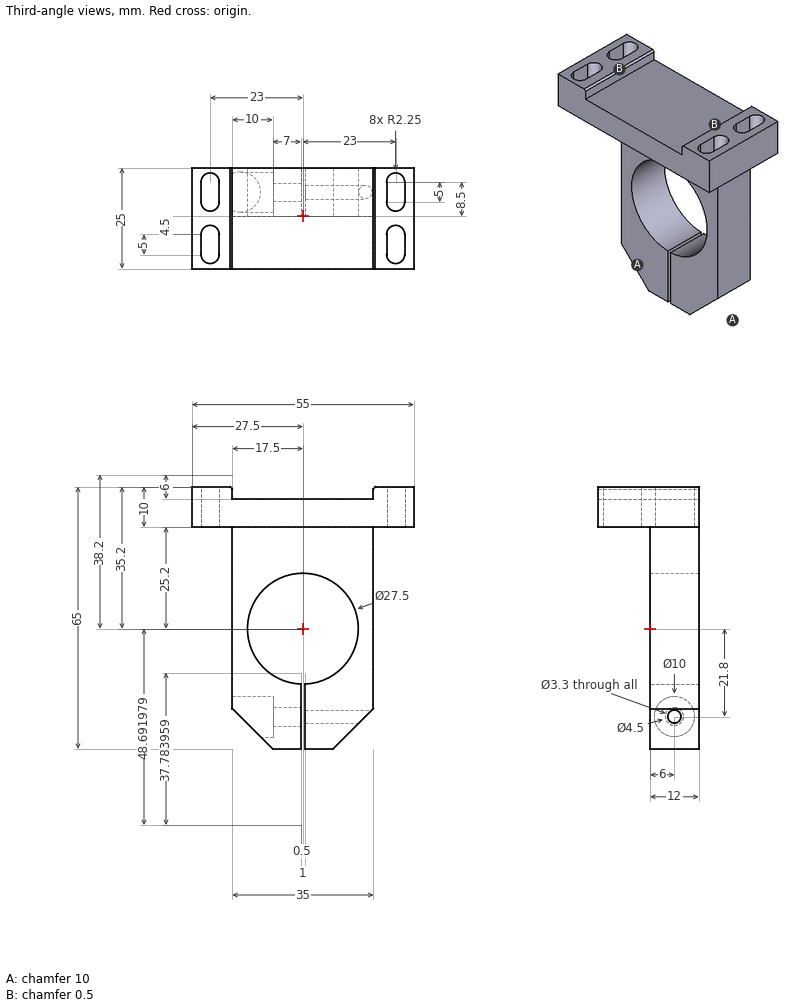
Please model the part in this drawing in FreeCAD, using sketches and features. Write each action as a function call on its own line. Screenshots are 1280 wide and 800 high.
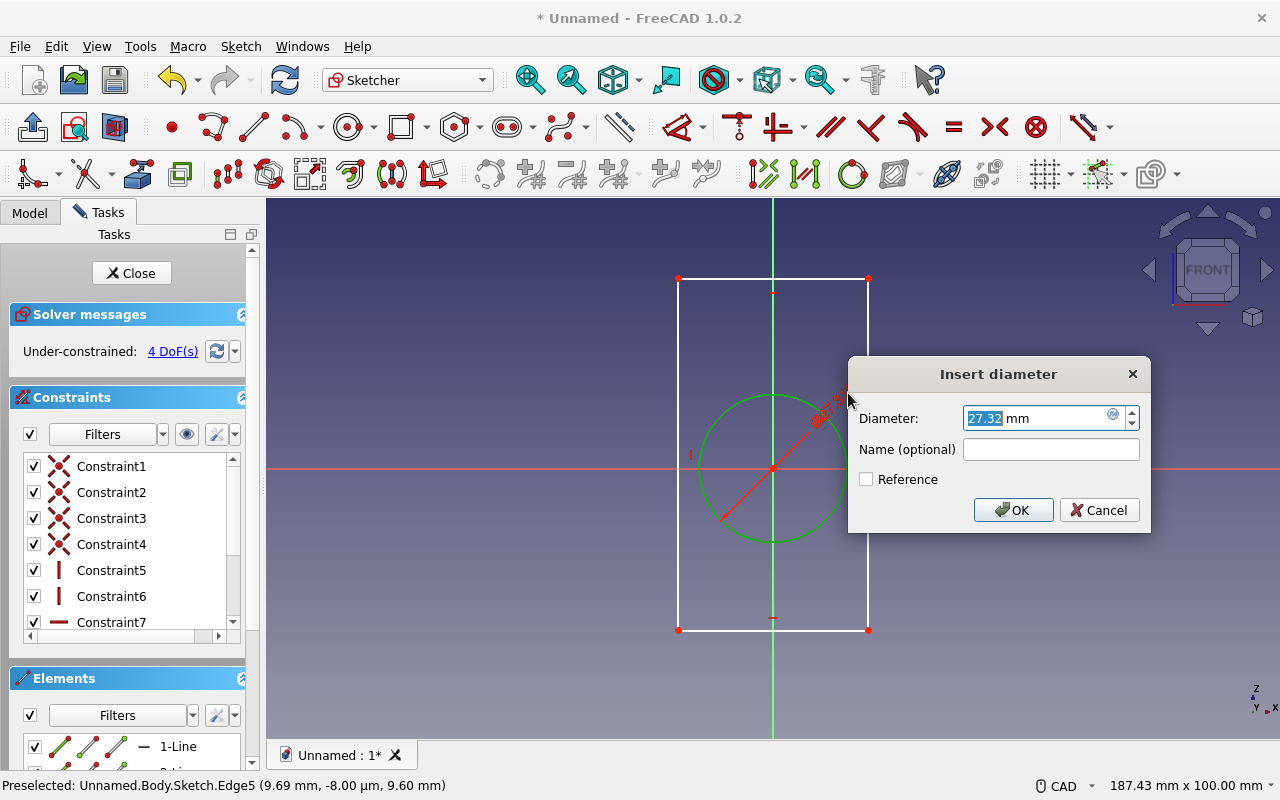
text(27.5)
key(Return)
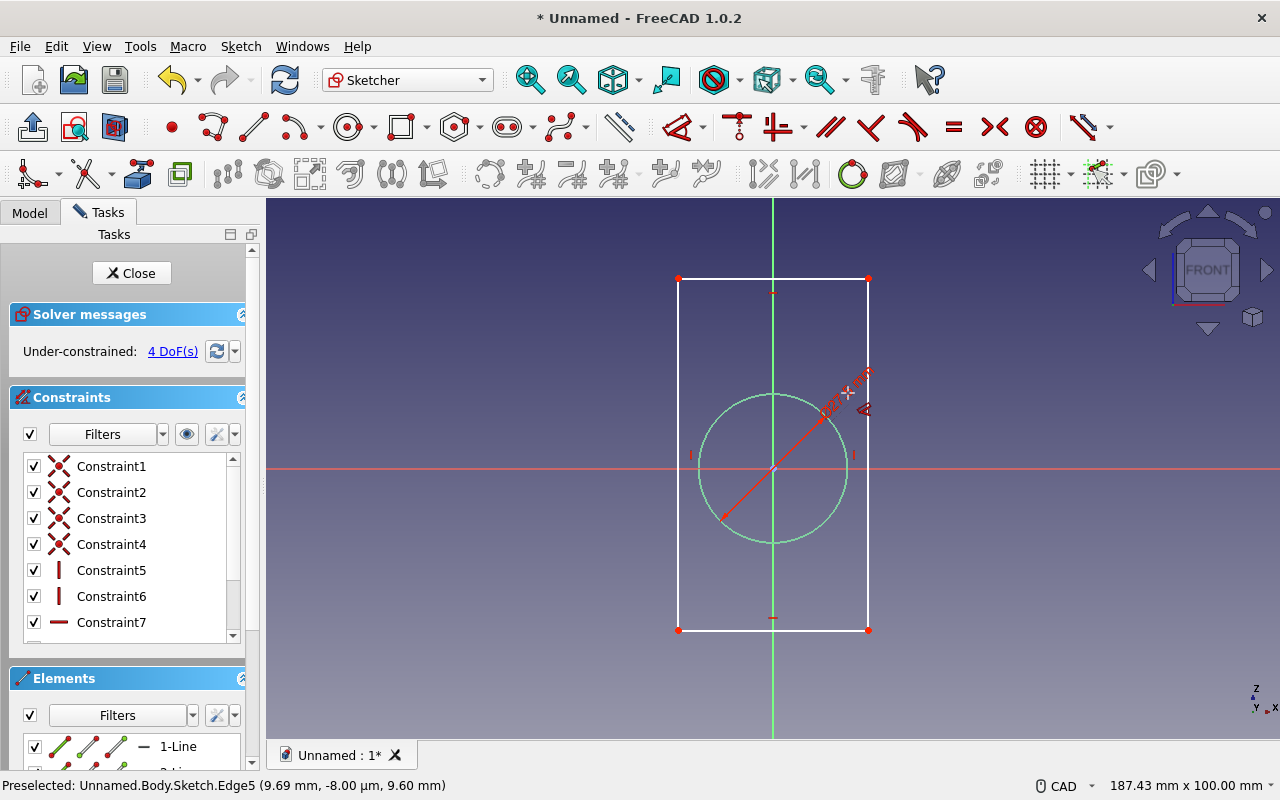
click(678, 385)
click(644, 455)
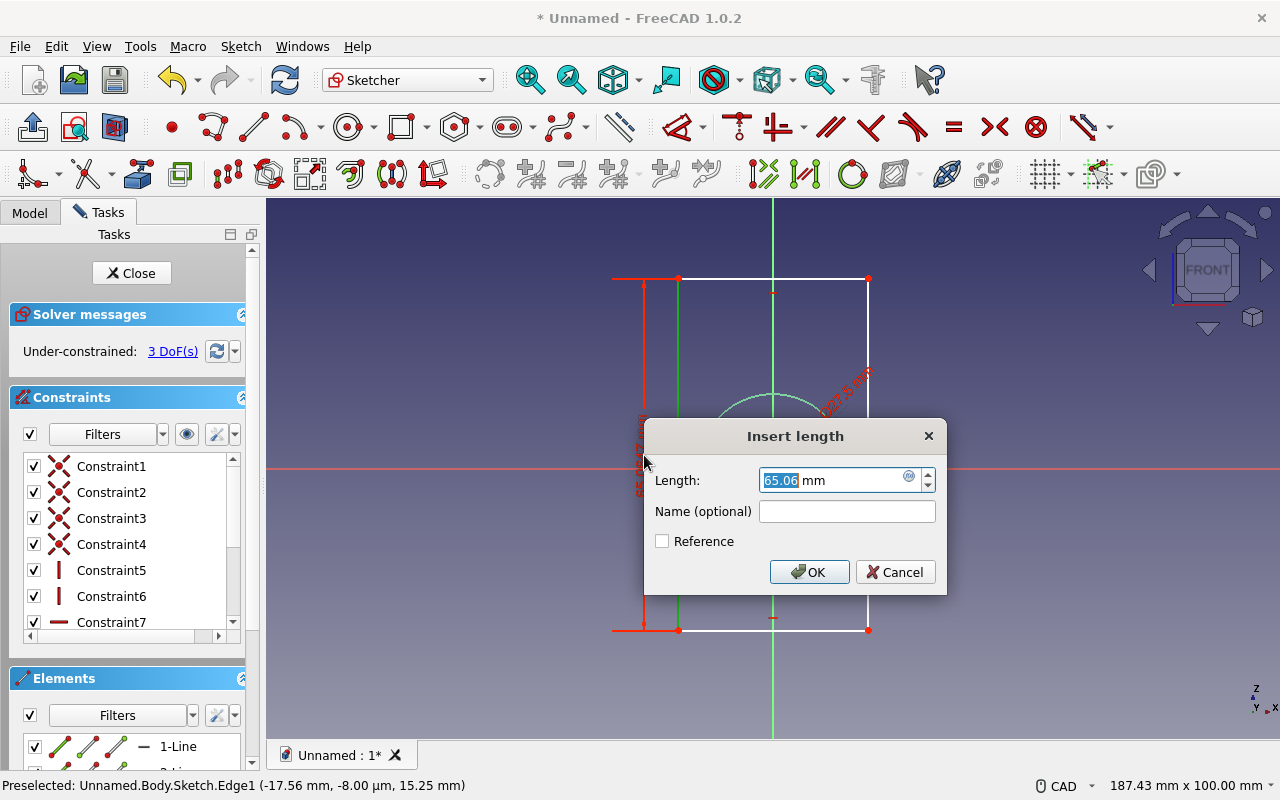
text(65)
key(Return)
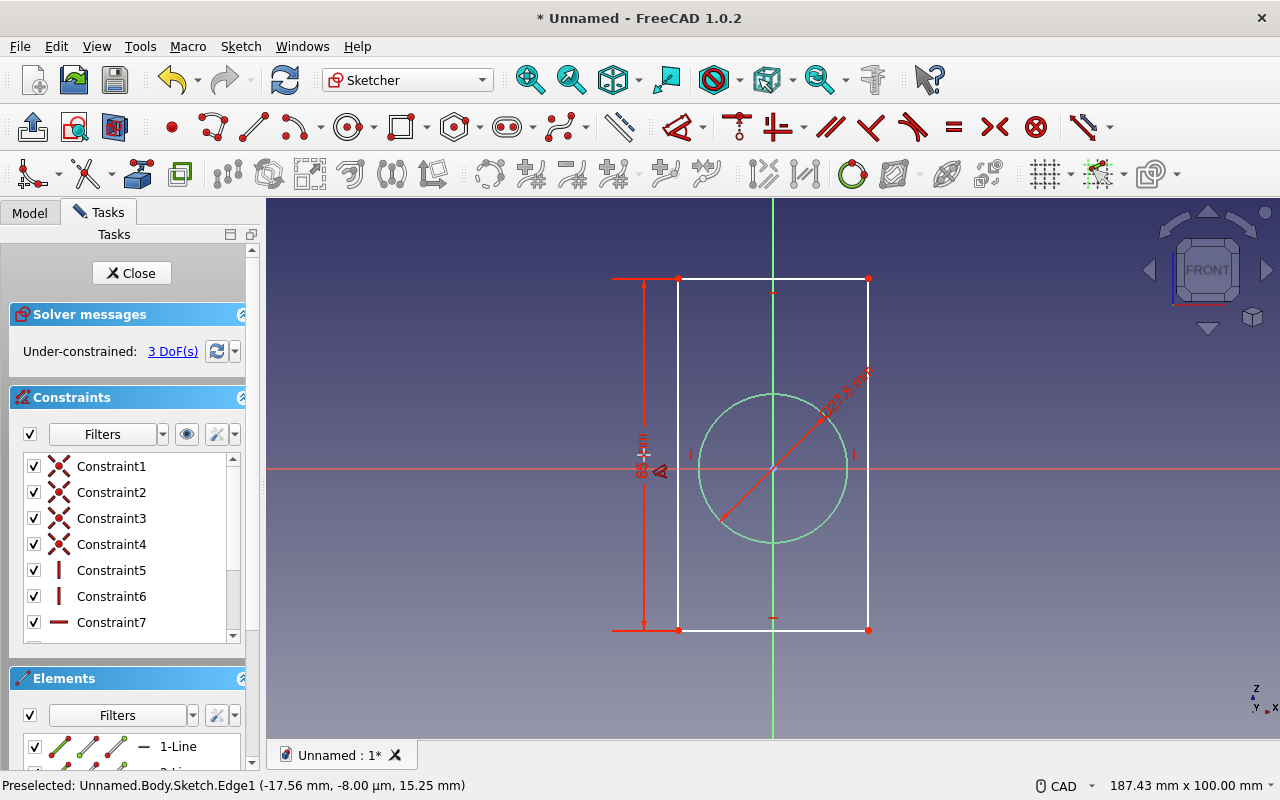
click(735, 631)
click(729, 665)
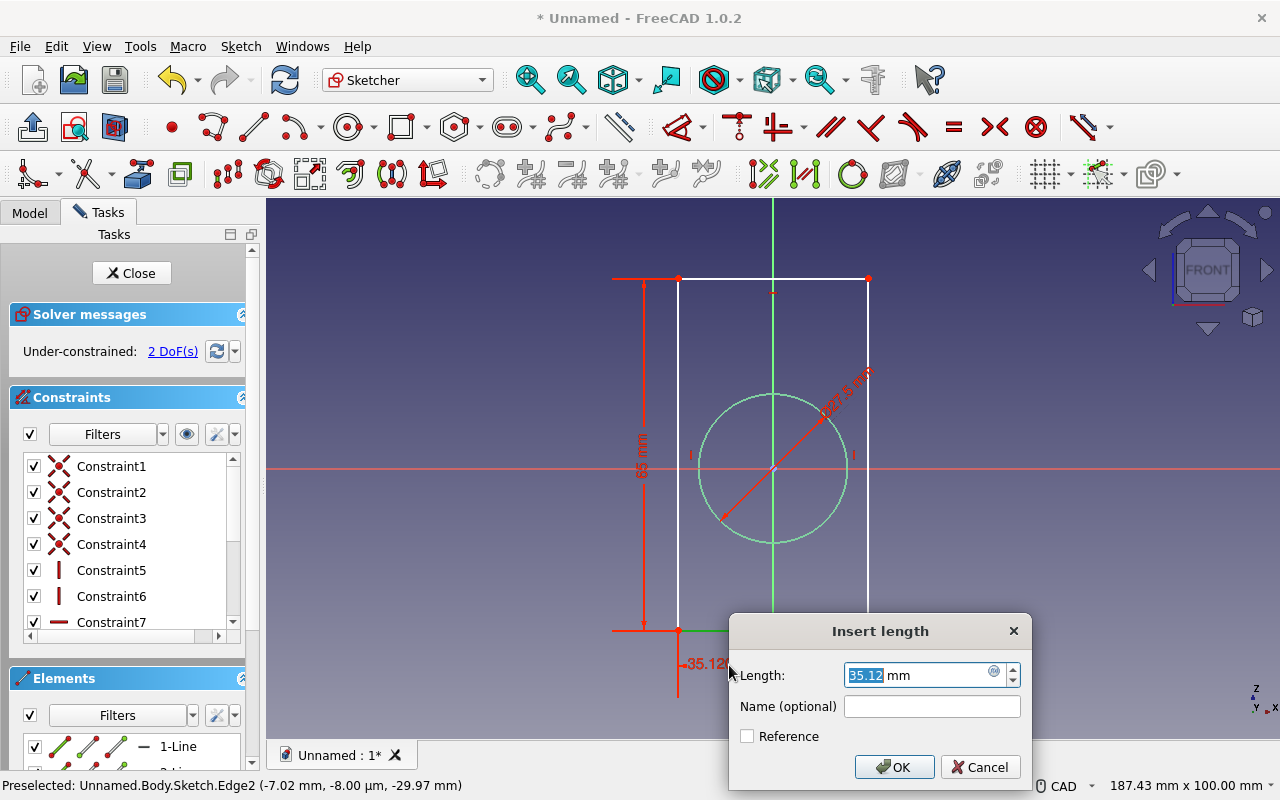
text(35)
key(Return)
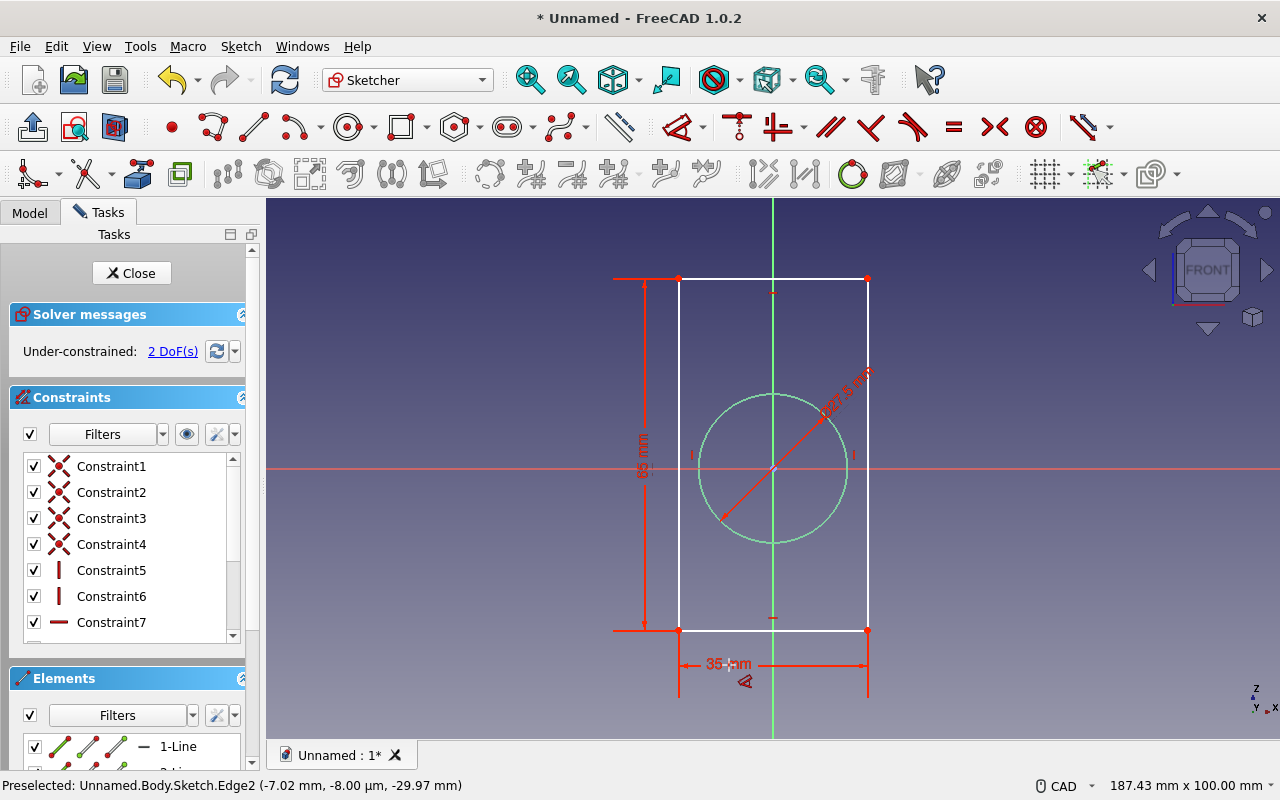
click(679, 279)
click(726, 245)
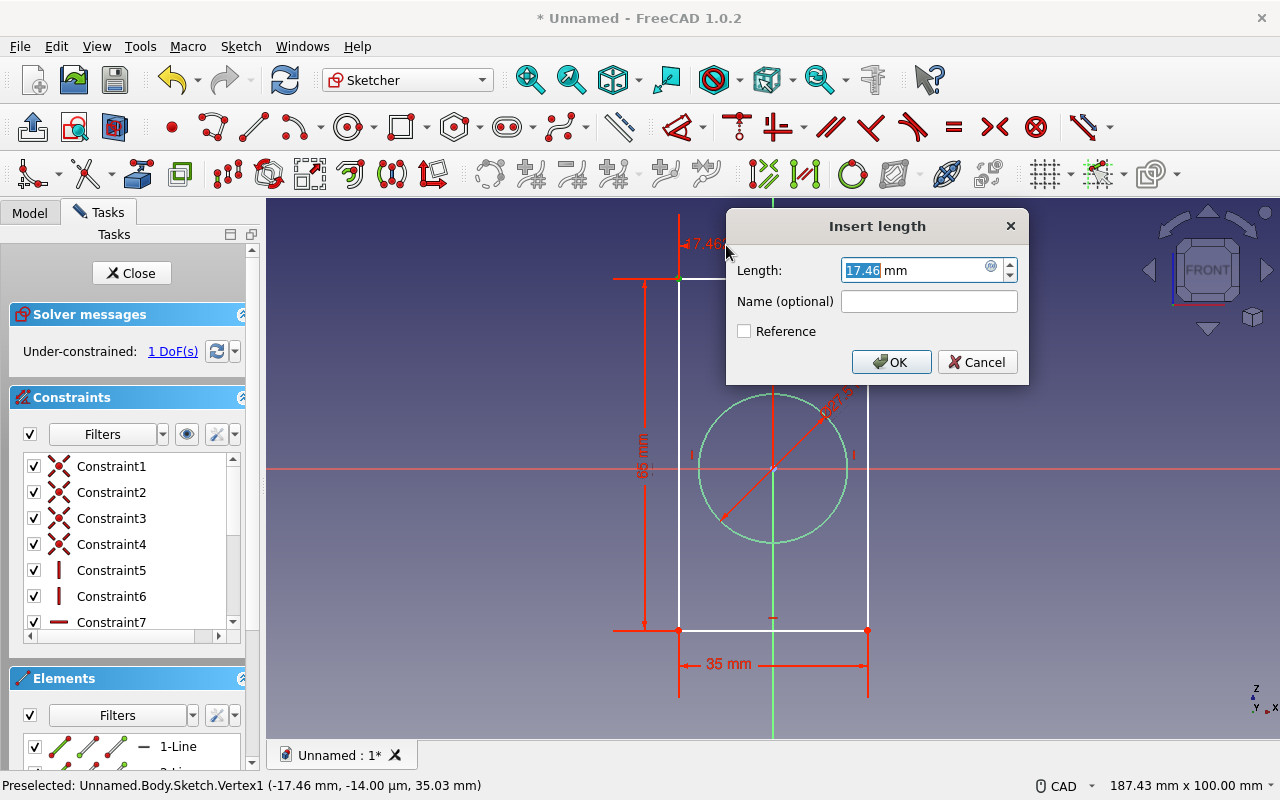
text(17.5)
key(Return)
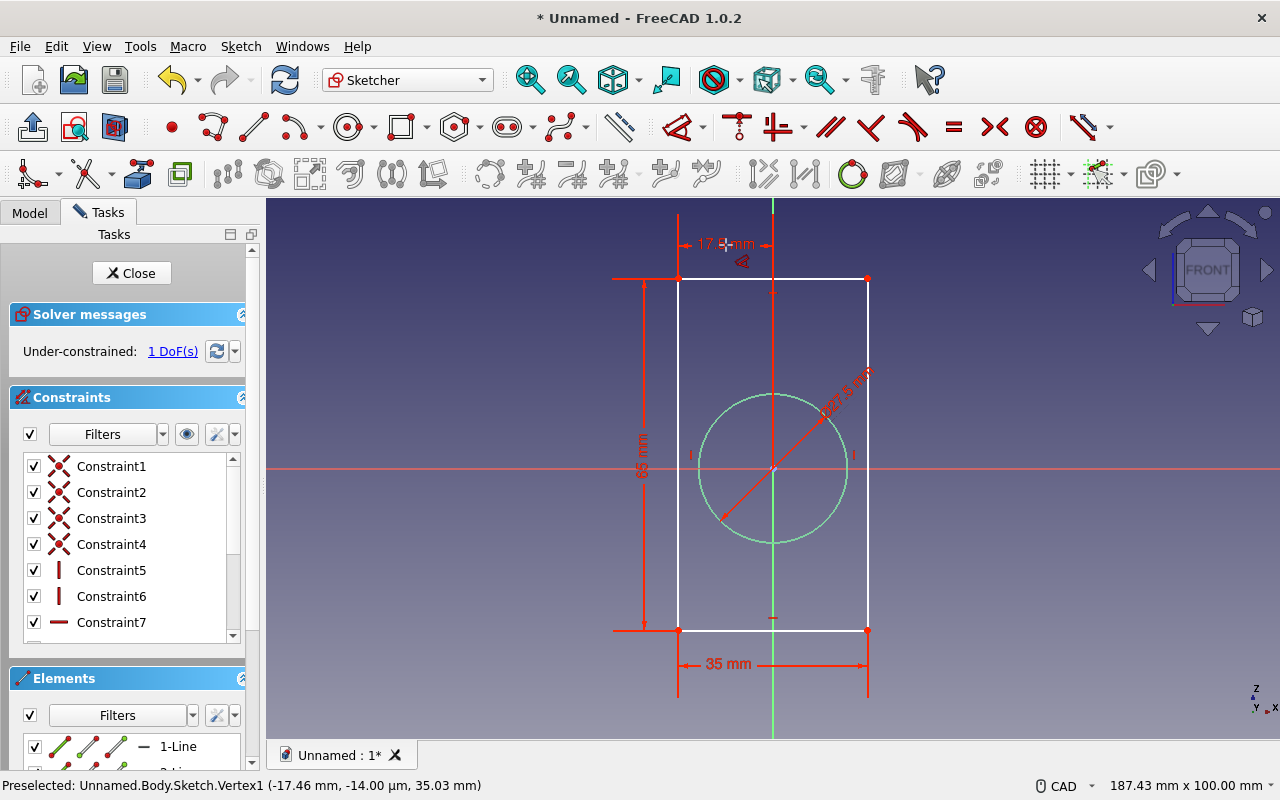
click(678, 279)
click(644, 374)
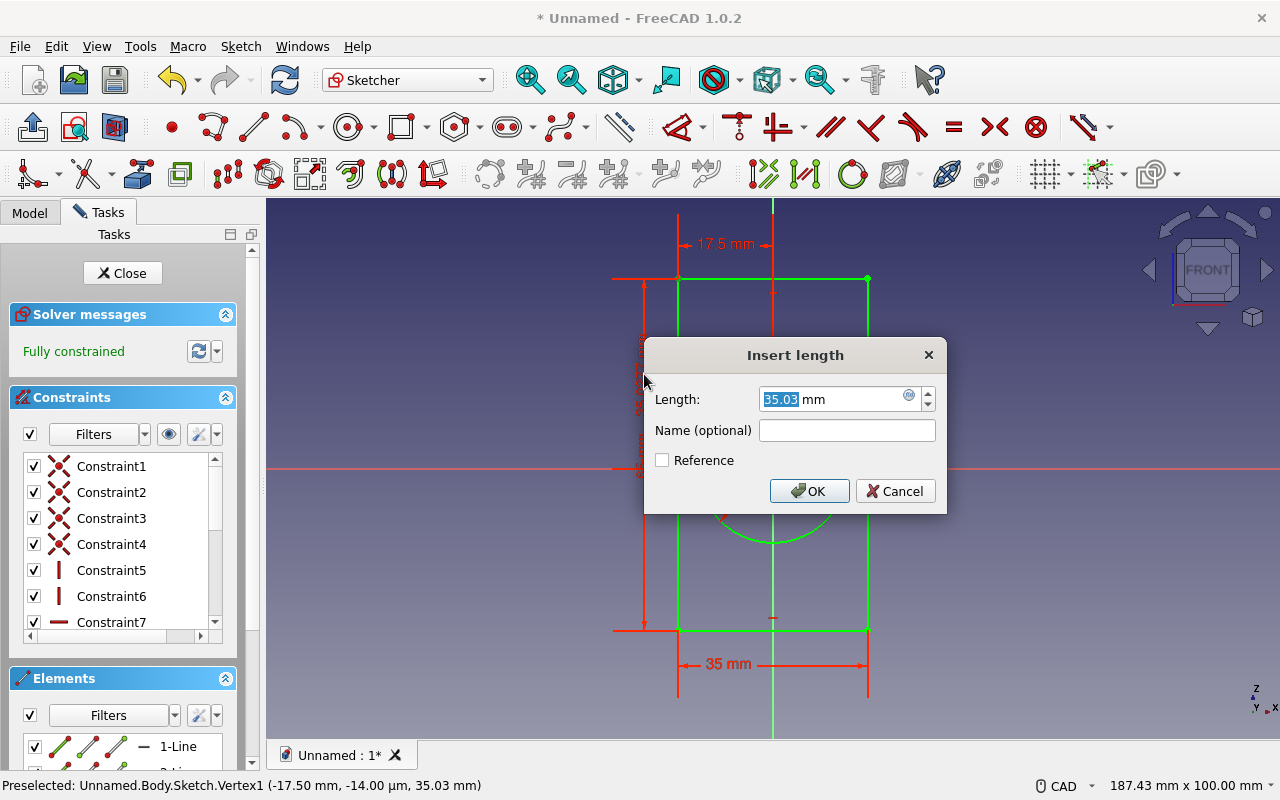
text(35.2)
key(Return)
key(Escape)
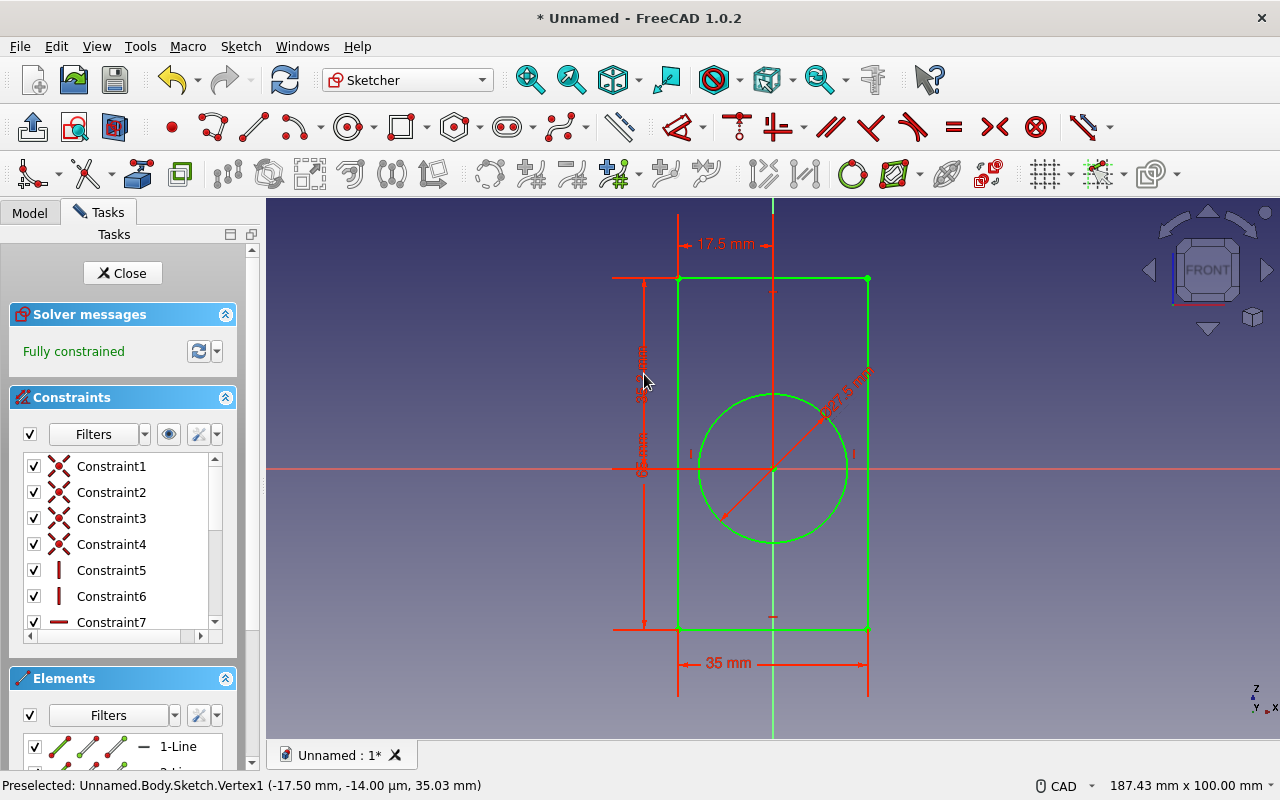
click(123, 273)